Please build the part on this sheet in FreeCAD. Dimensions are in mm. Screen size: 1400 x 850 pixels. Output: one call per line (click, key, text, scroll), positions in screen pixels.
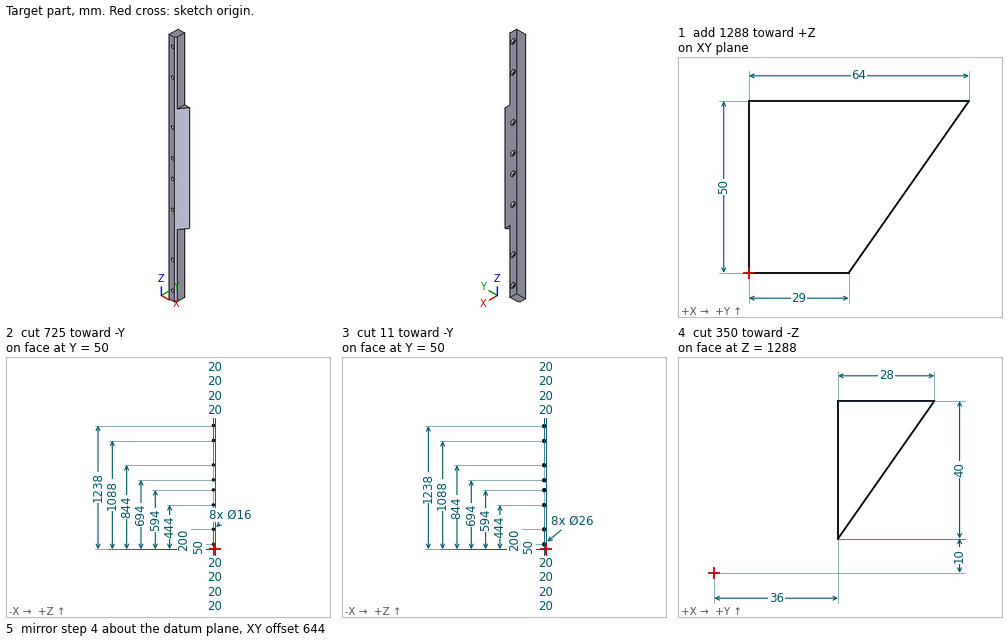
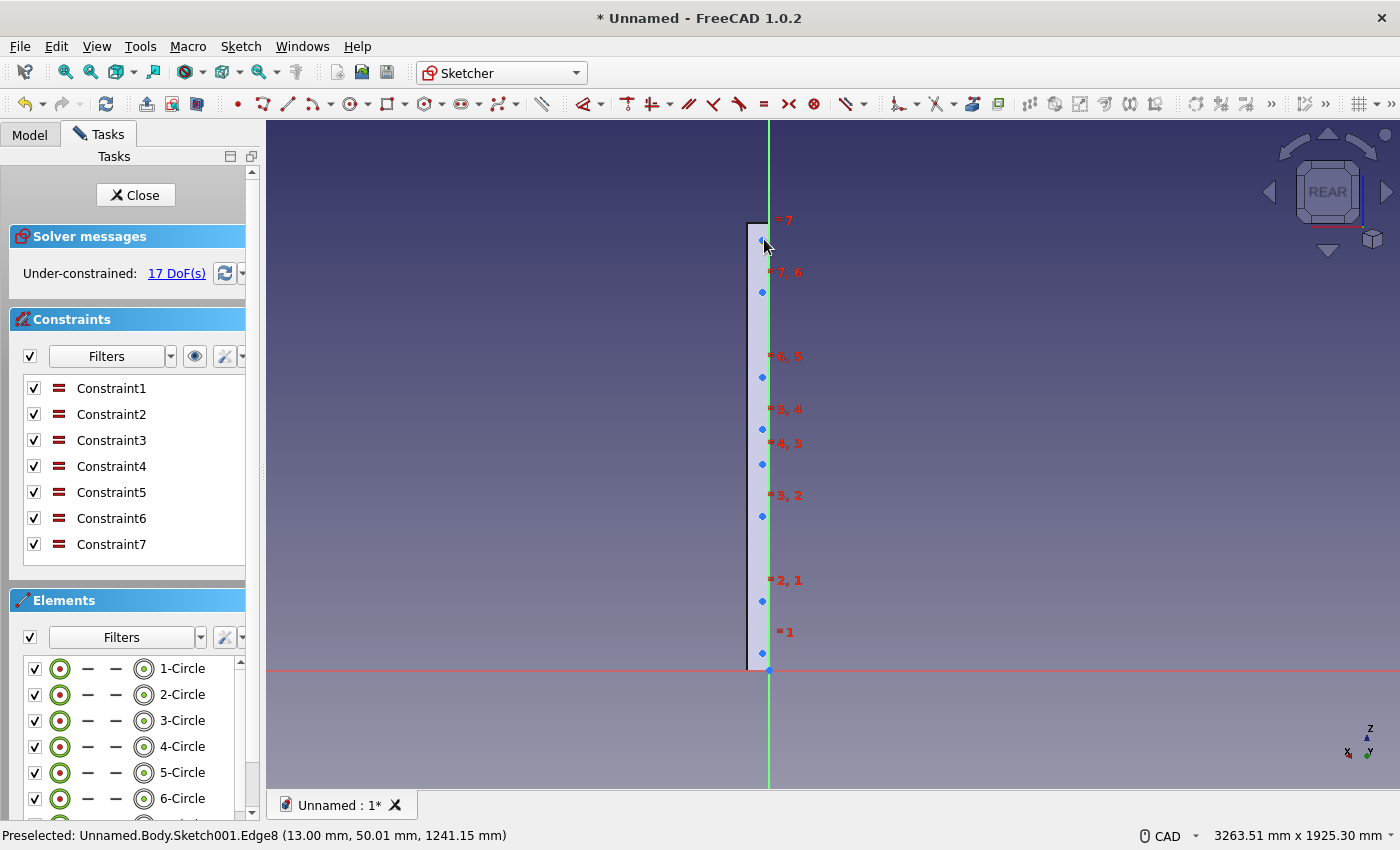
scroll(764, 652, up, 10)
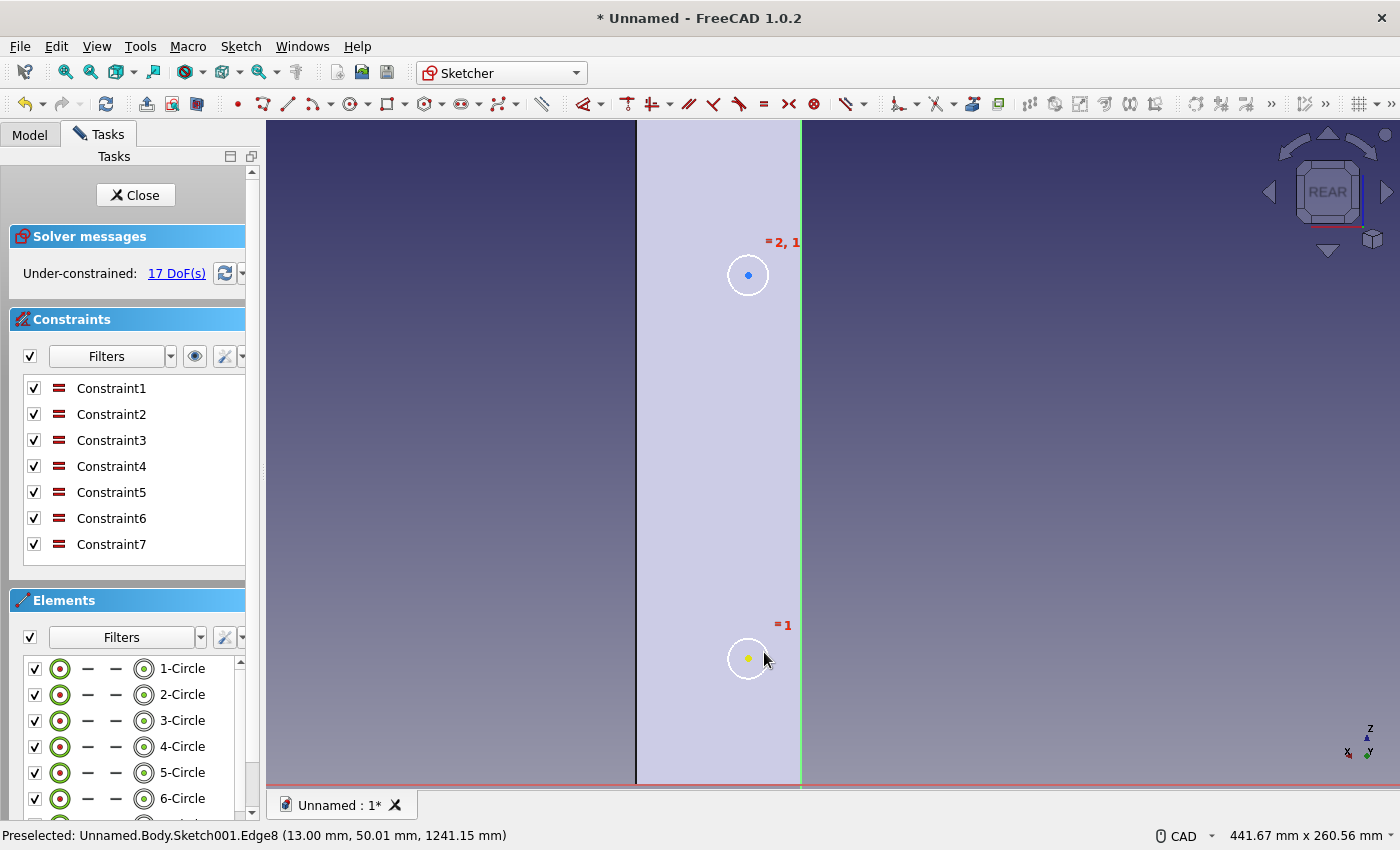
click(762, 645)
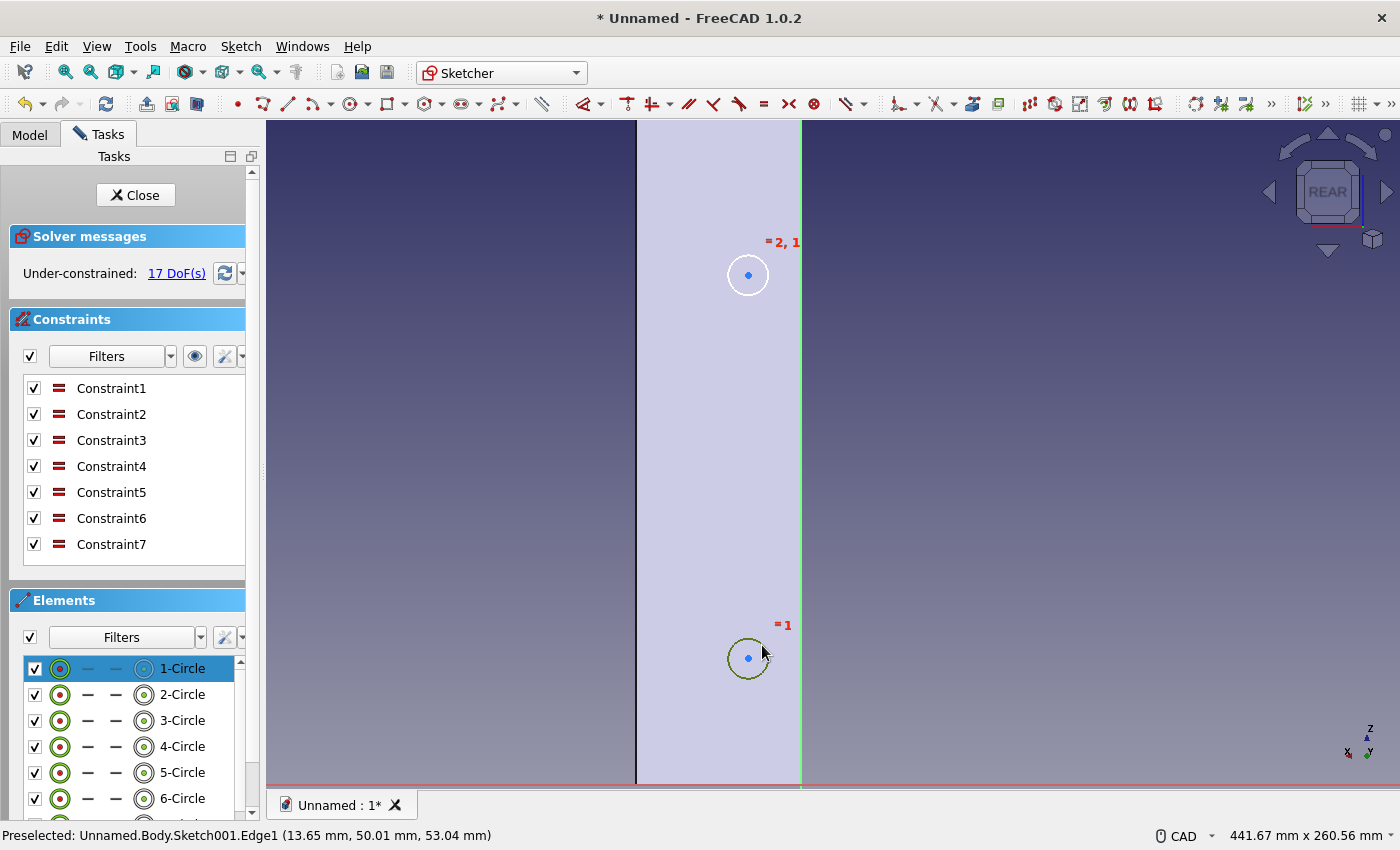
key(k)
key(o)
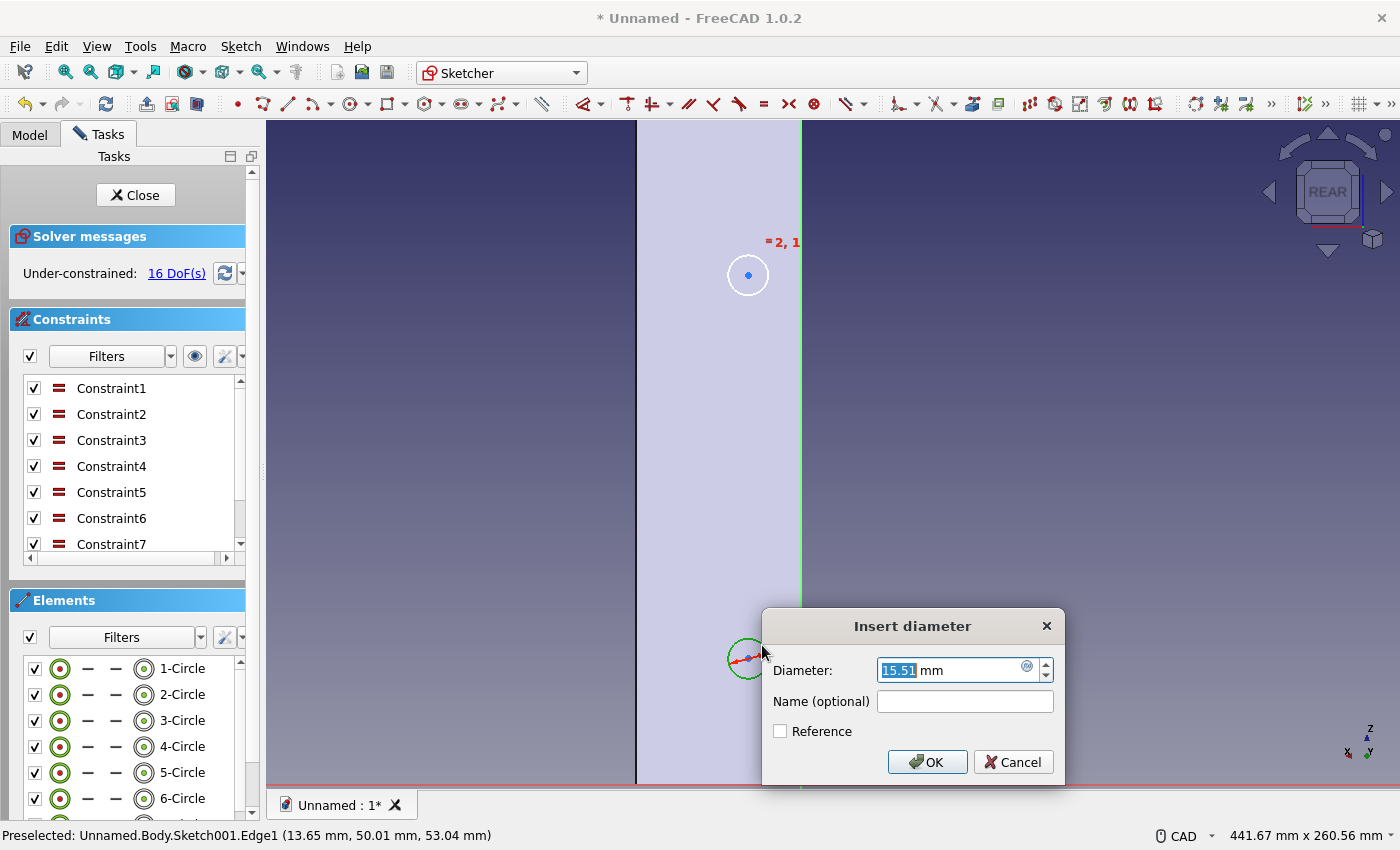
text(16)
key(Return)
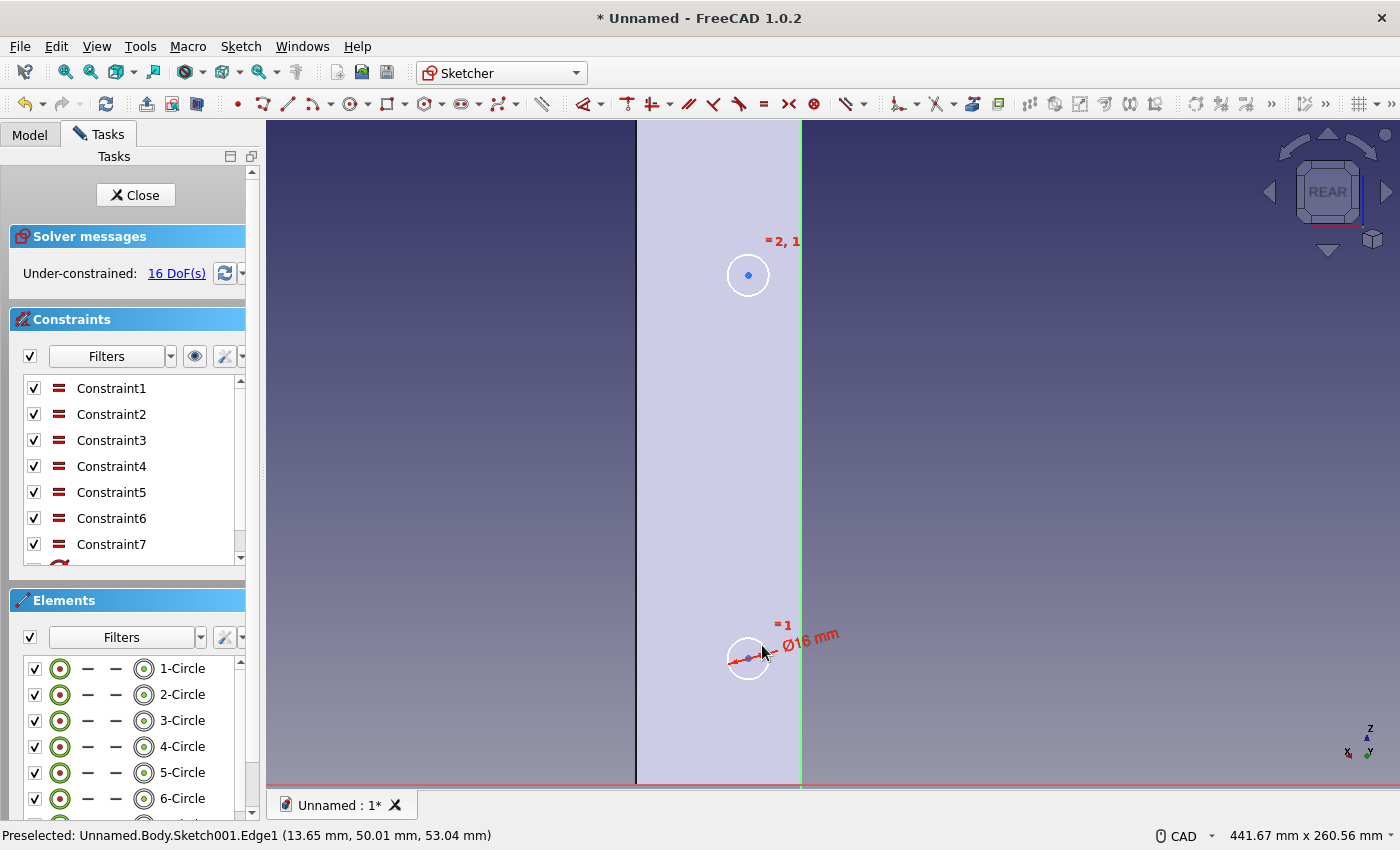
click(748, 659)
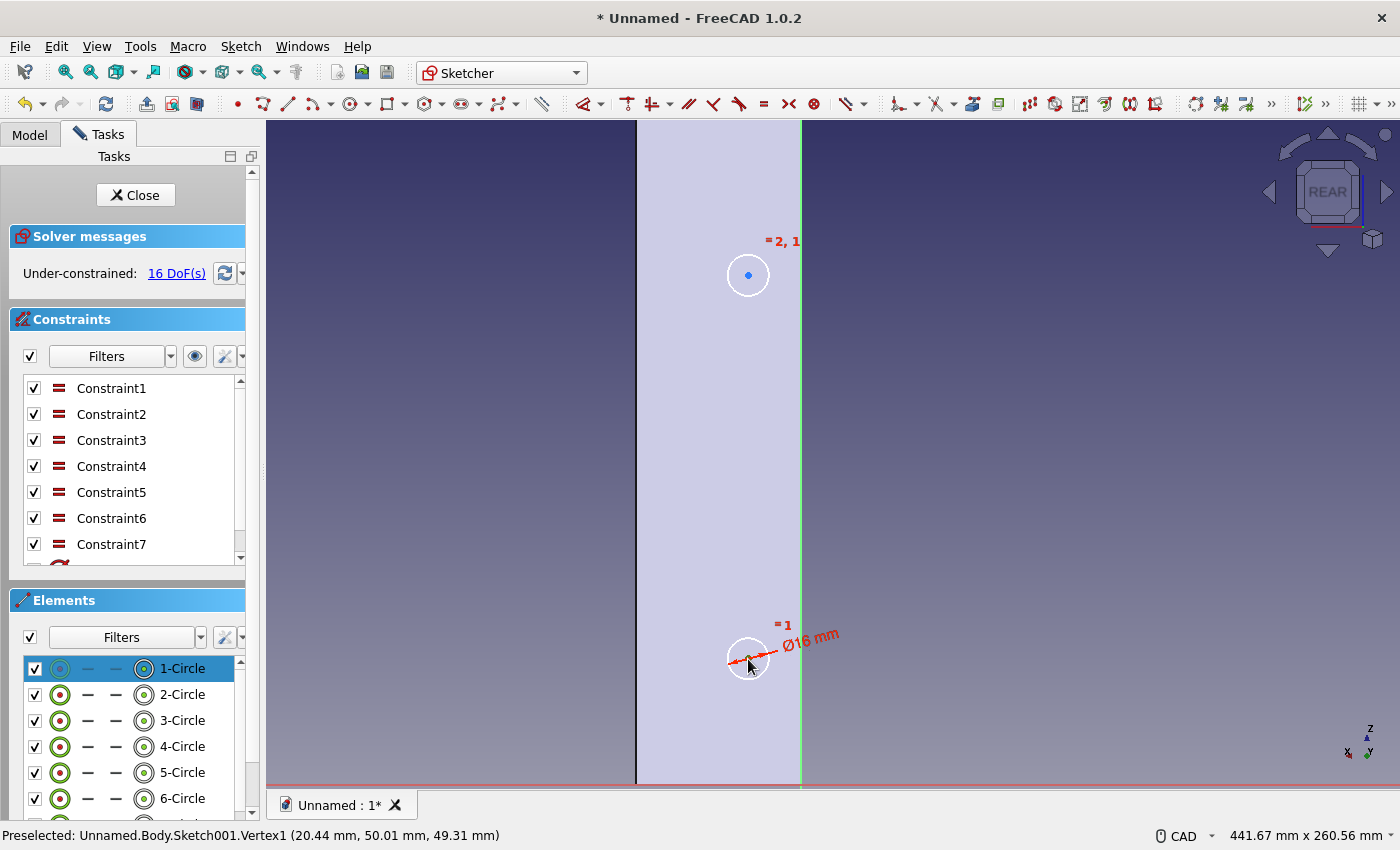
key(l)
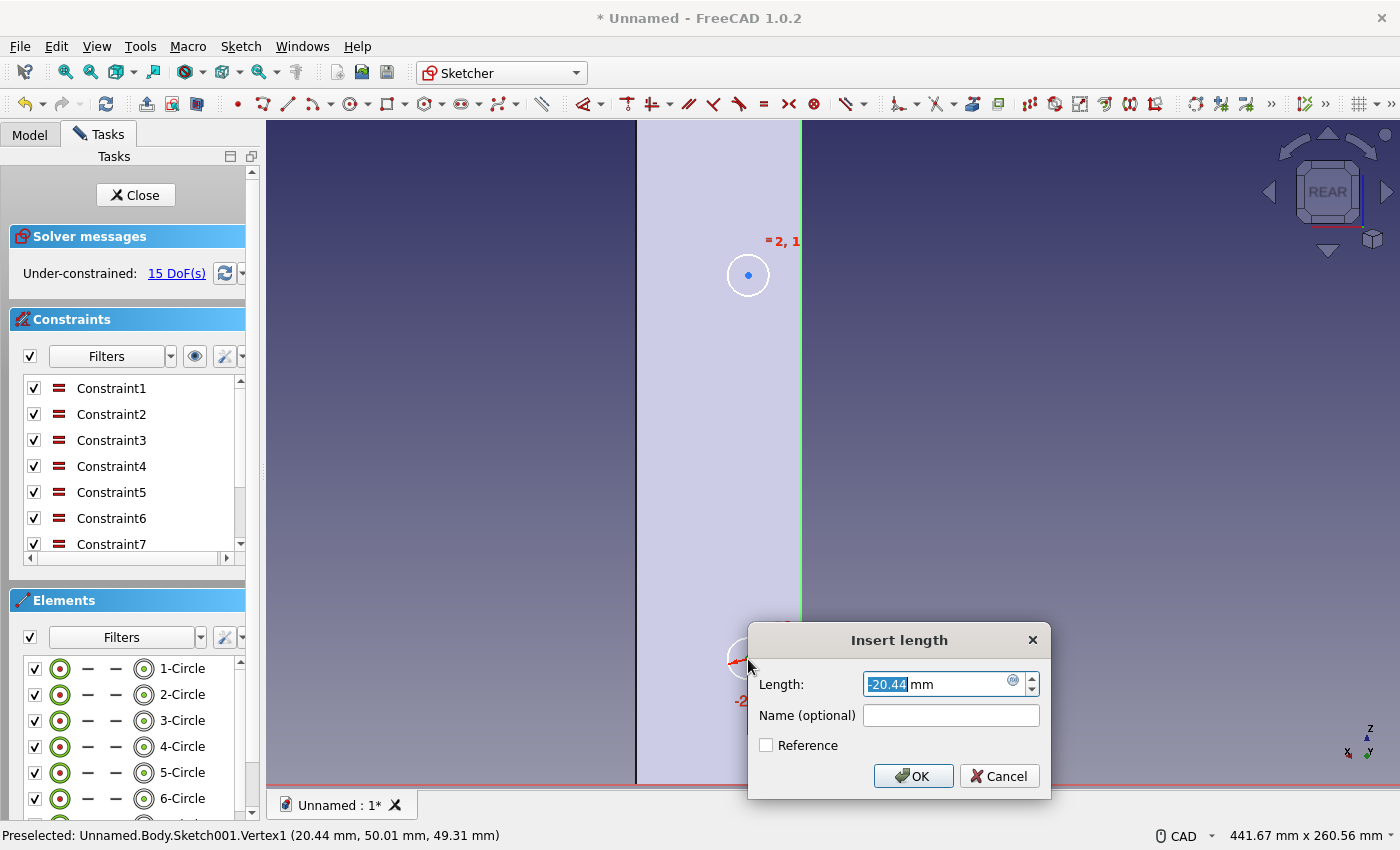
text(-20)
key(Return)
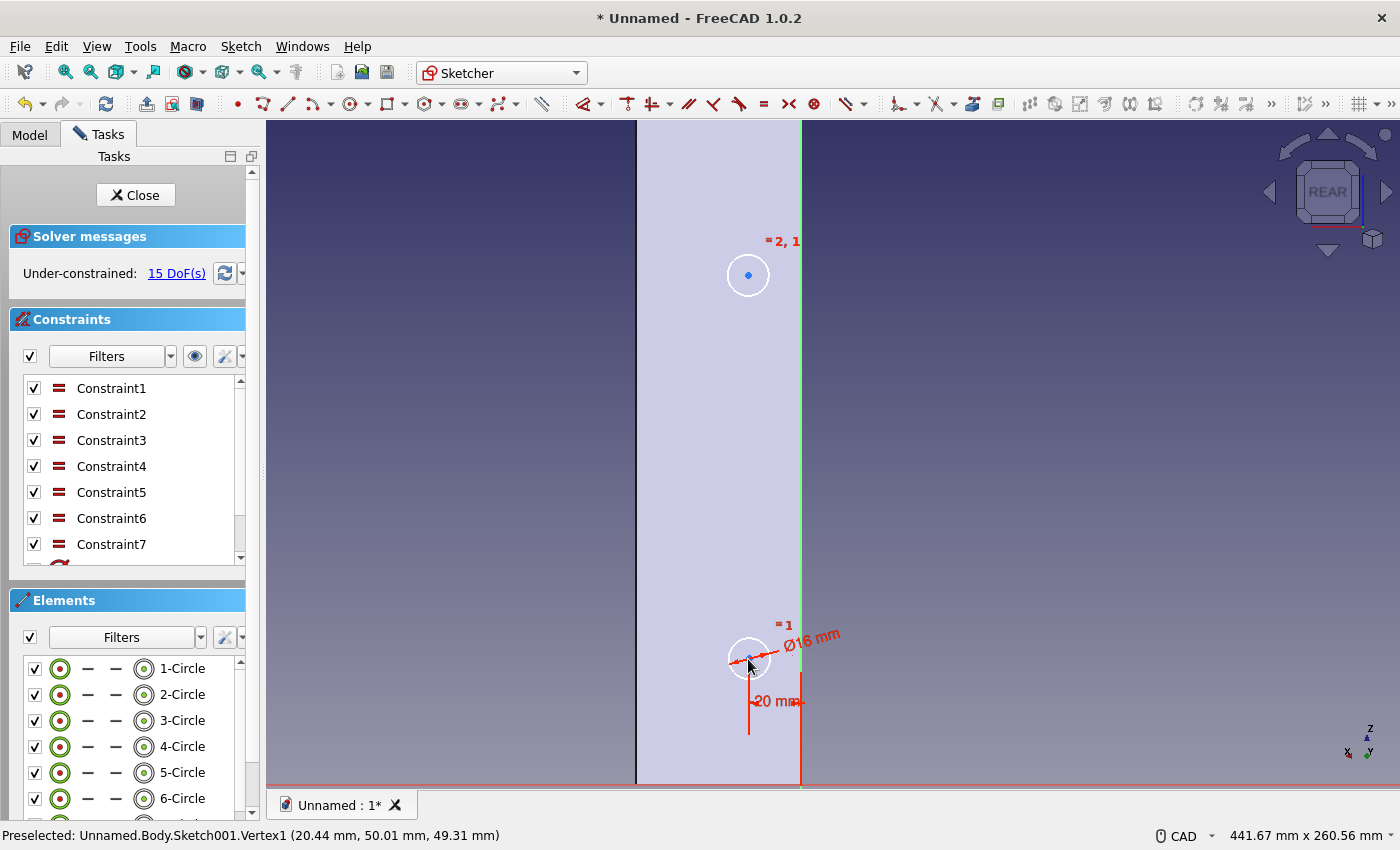
scroll(764, 653, down, 10)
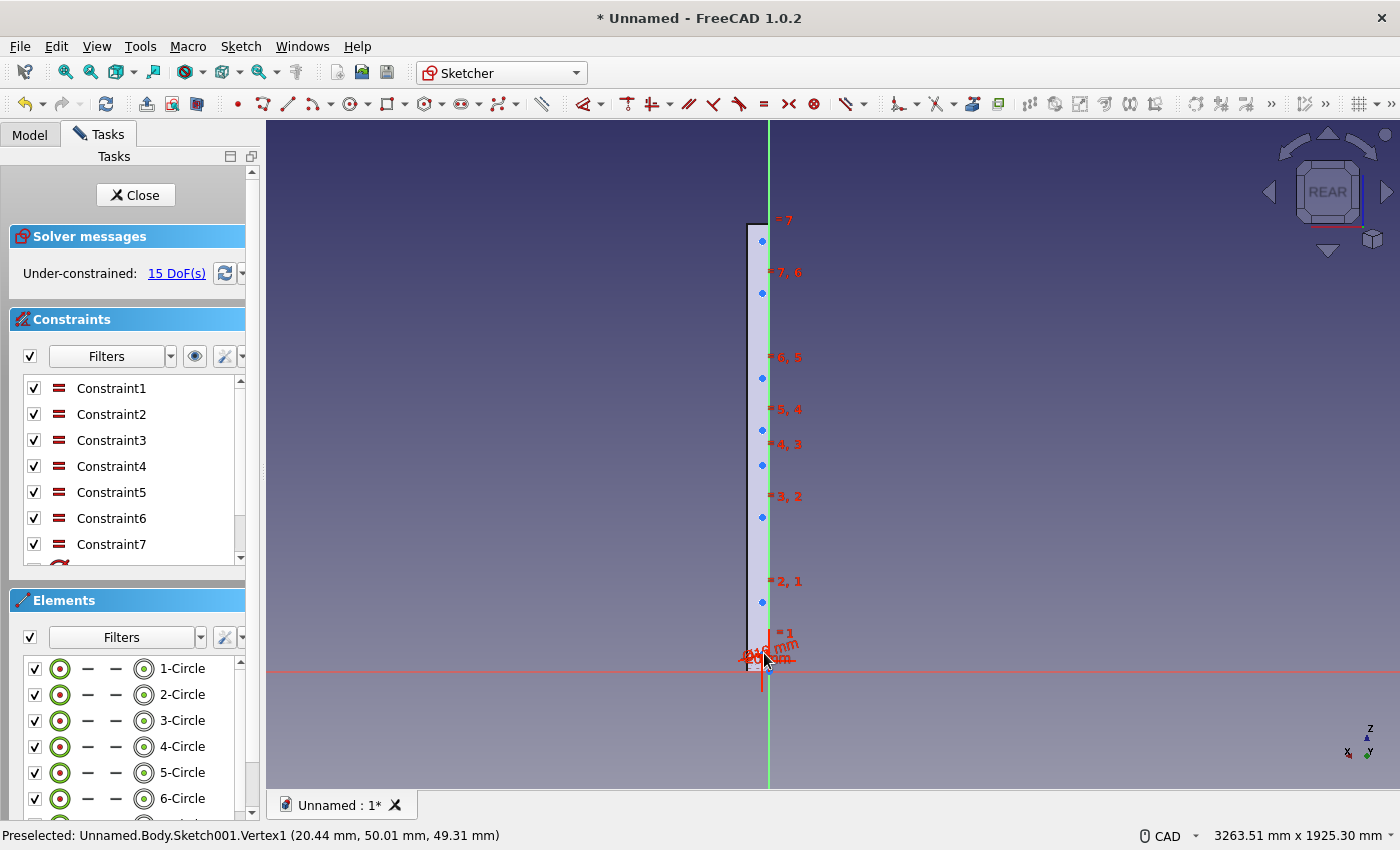
scroll(762, 654, up, 5)